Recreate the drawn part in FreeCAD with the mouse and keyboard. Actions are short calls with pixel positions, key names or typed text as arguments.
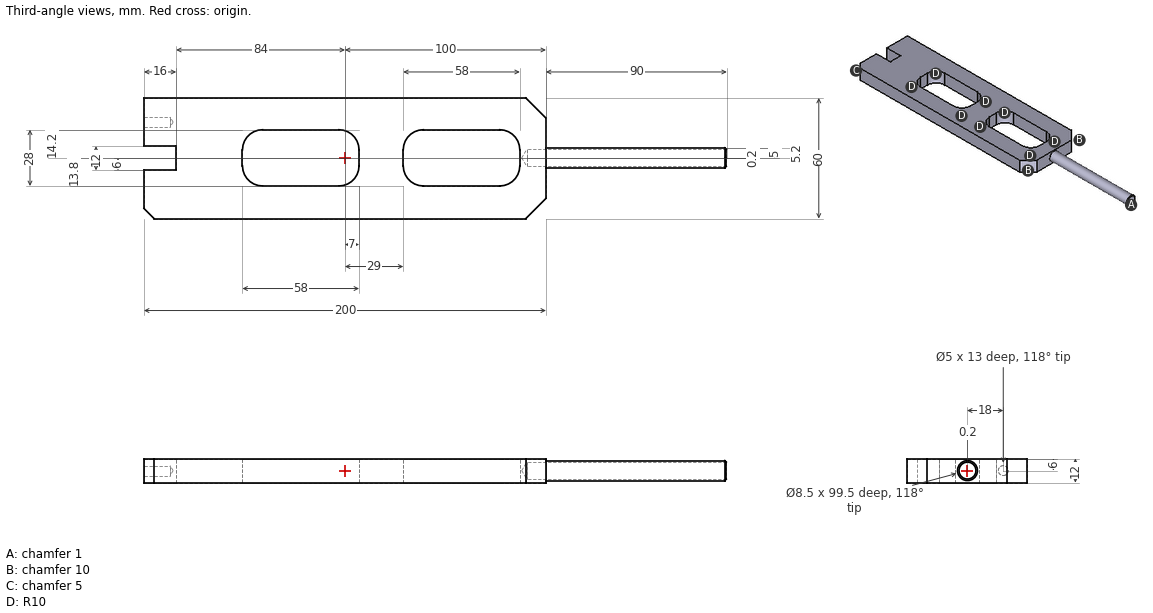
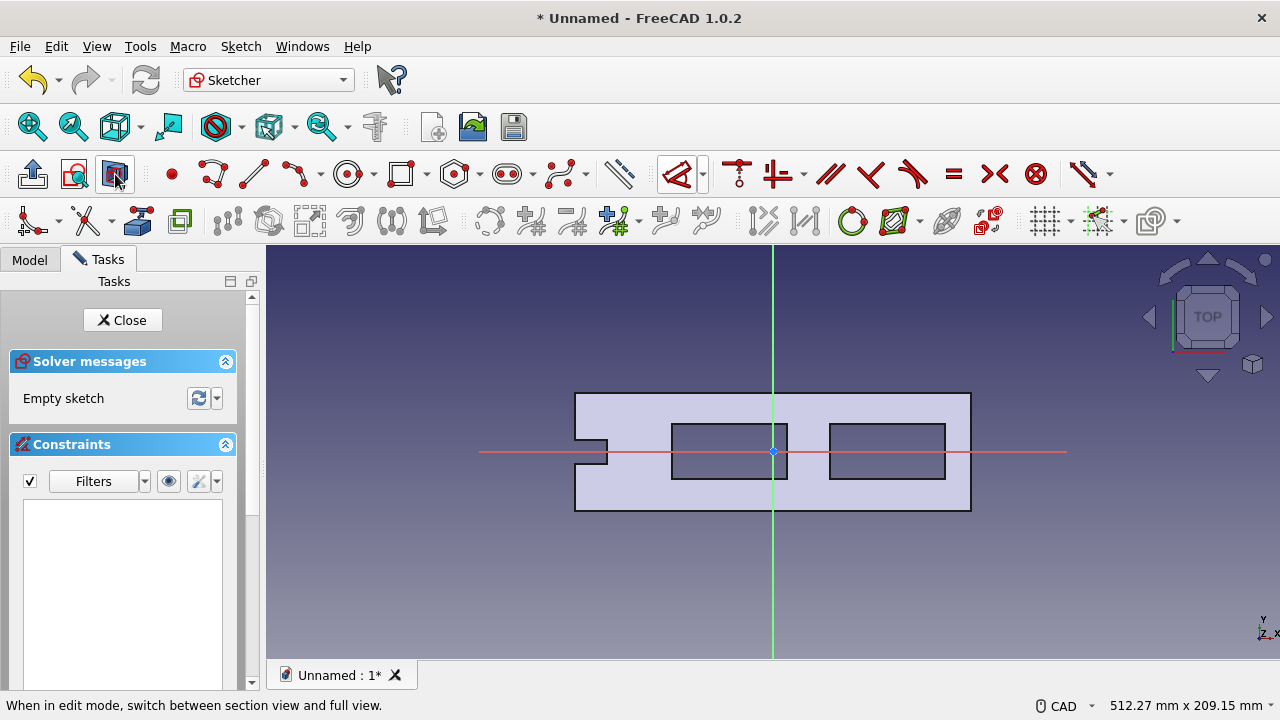
scroll(294, 475, down, 1)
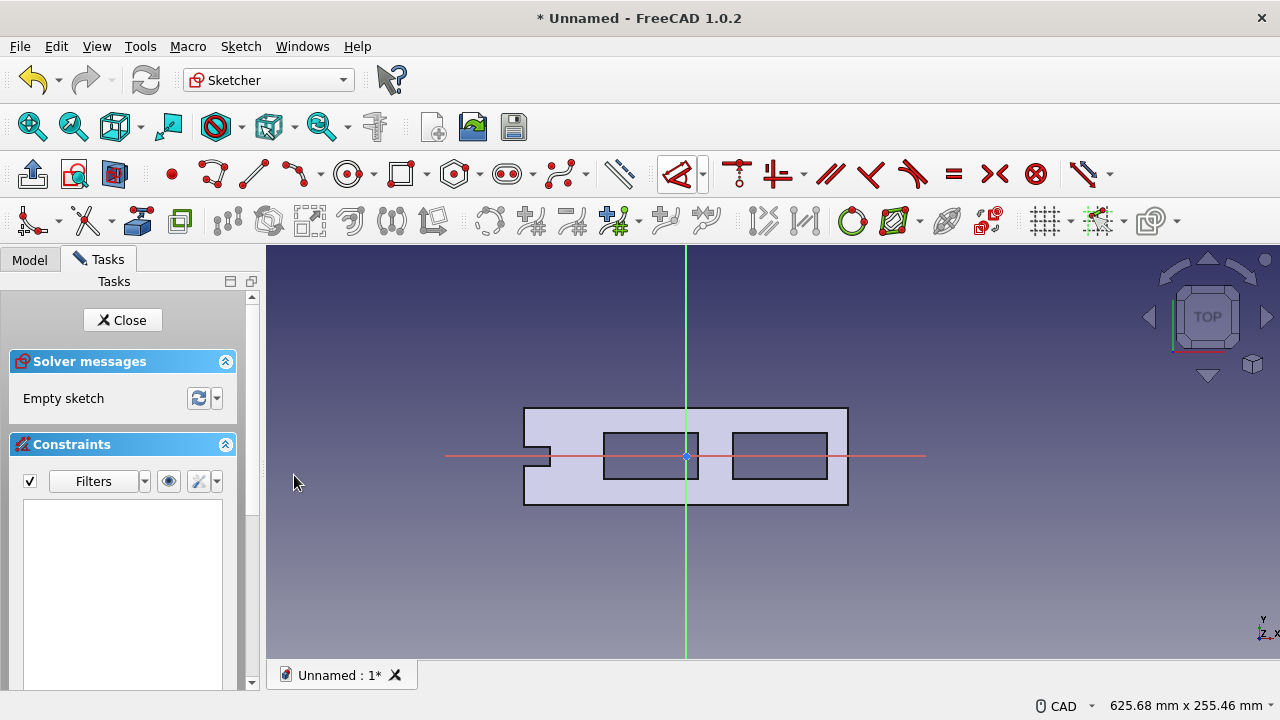
scroll(1005, 452, up, 3)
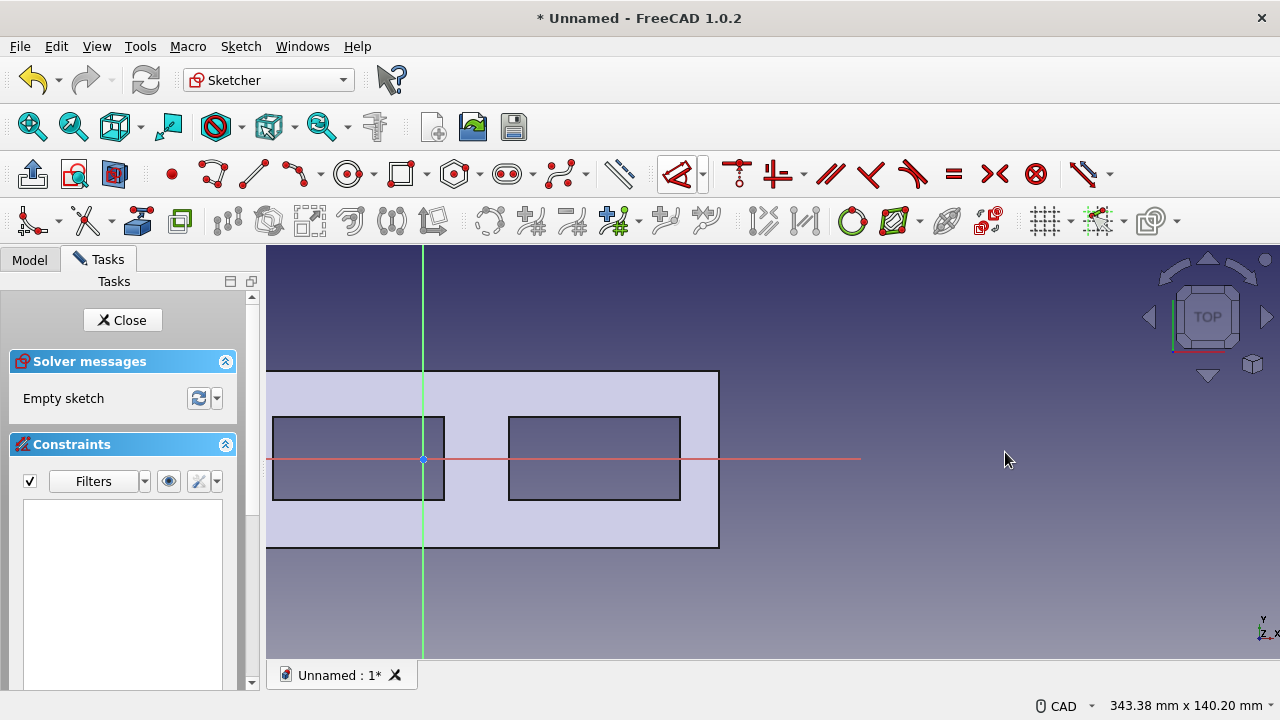
key(g)
key(r)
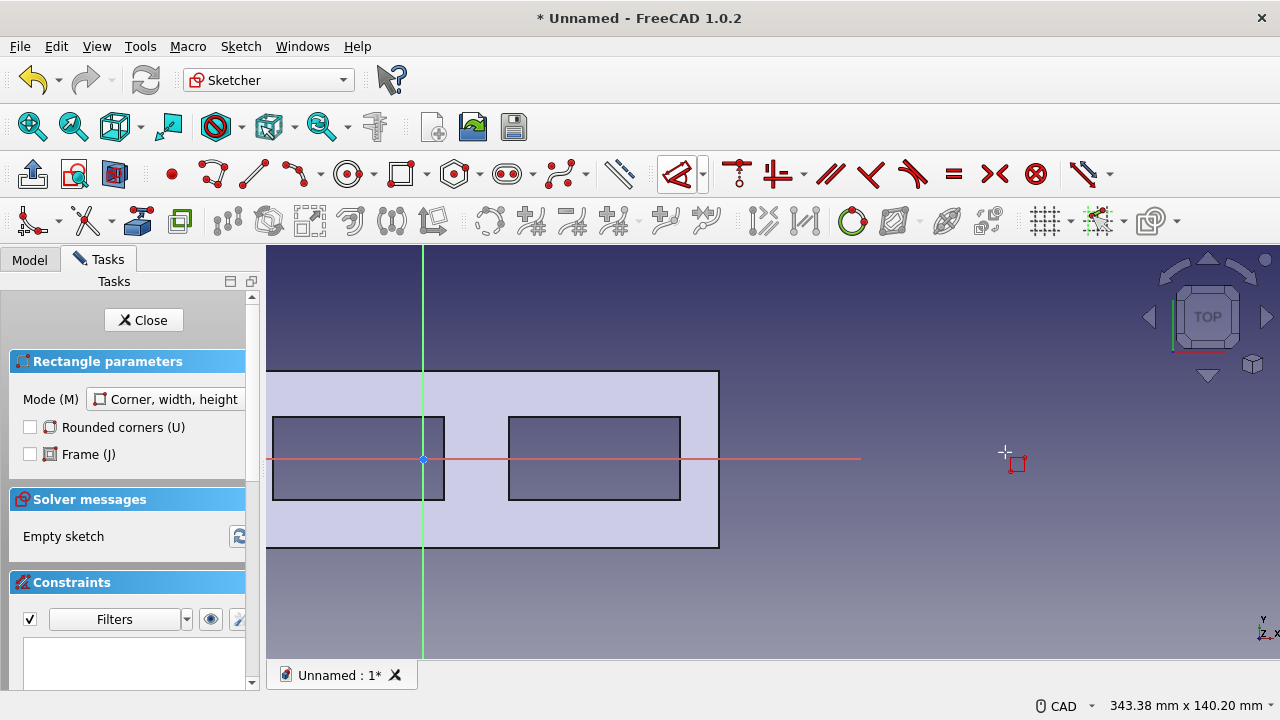
click(719, 444)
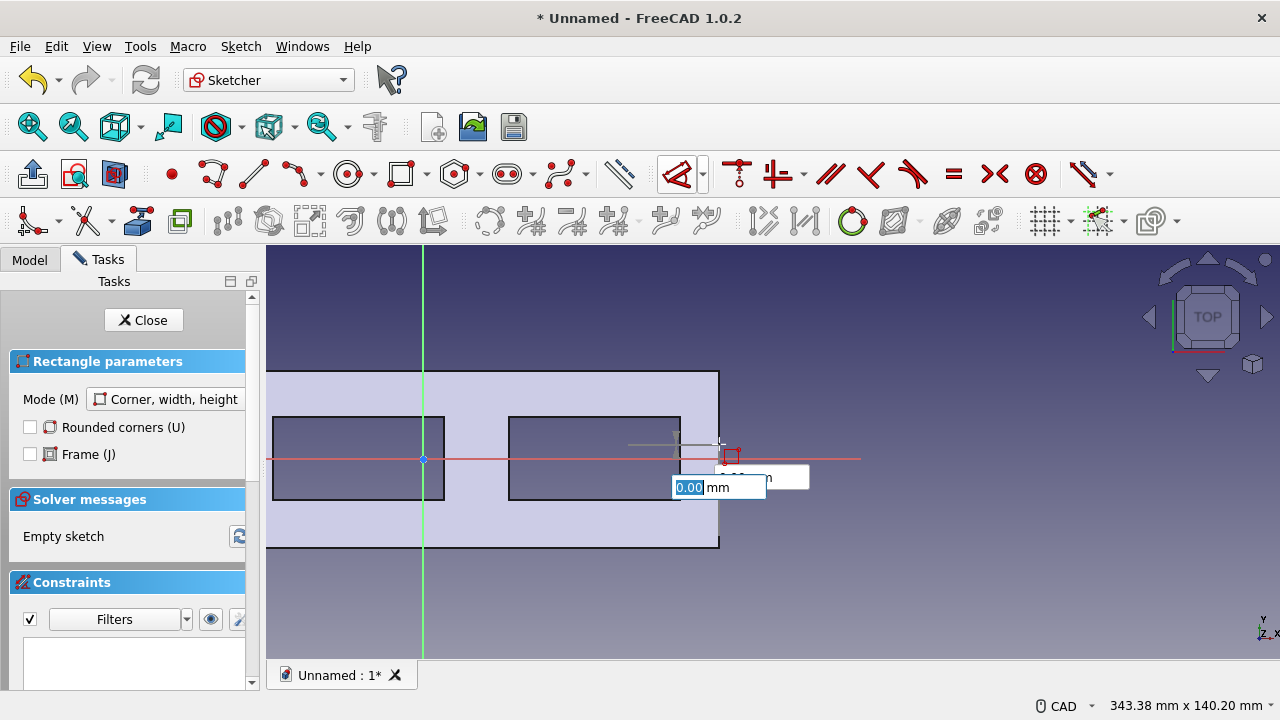
scroll(985, 459, up, 17)
move(950, 437)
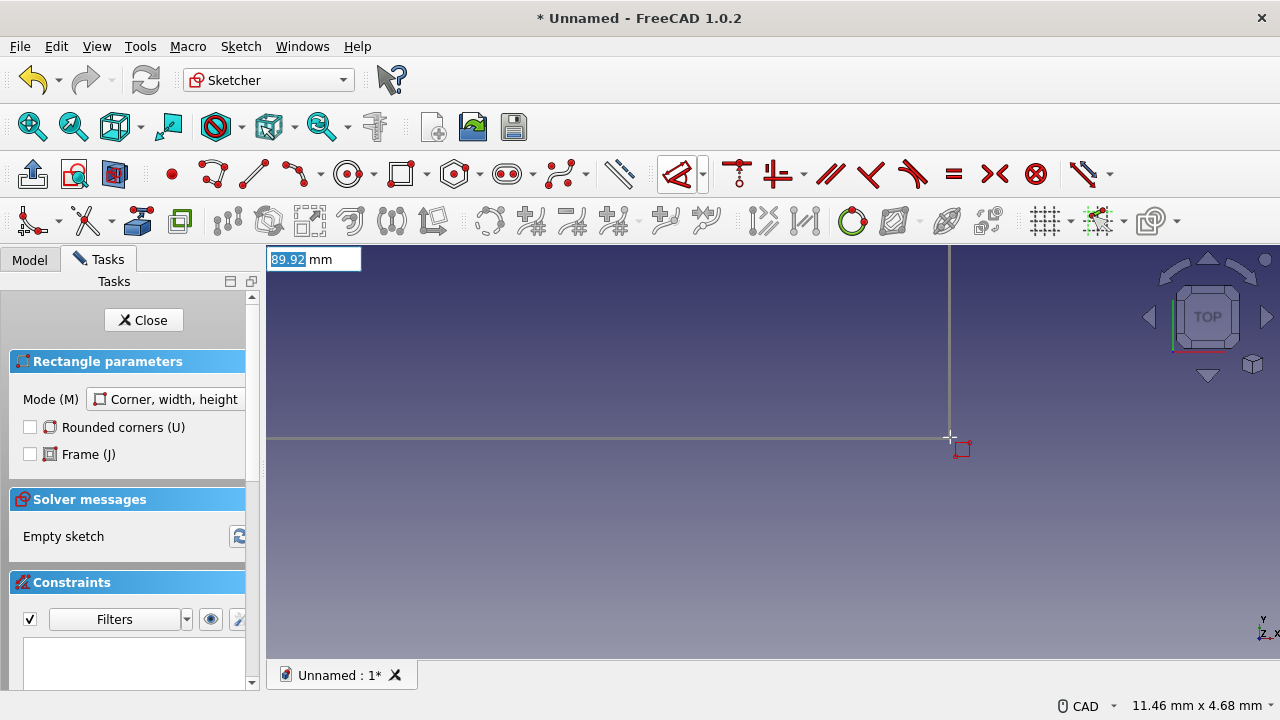
text(90)
key(Tab)
text(5)
key(Return)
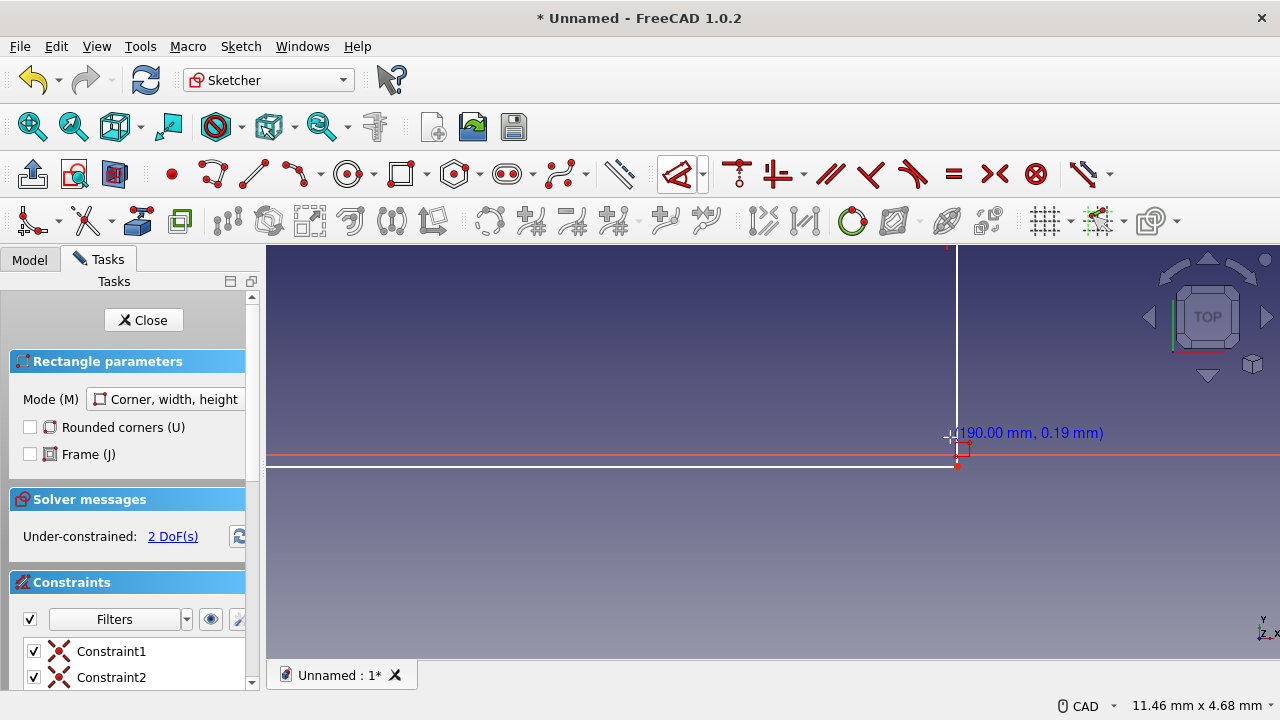
click(254, 174)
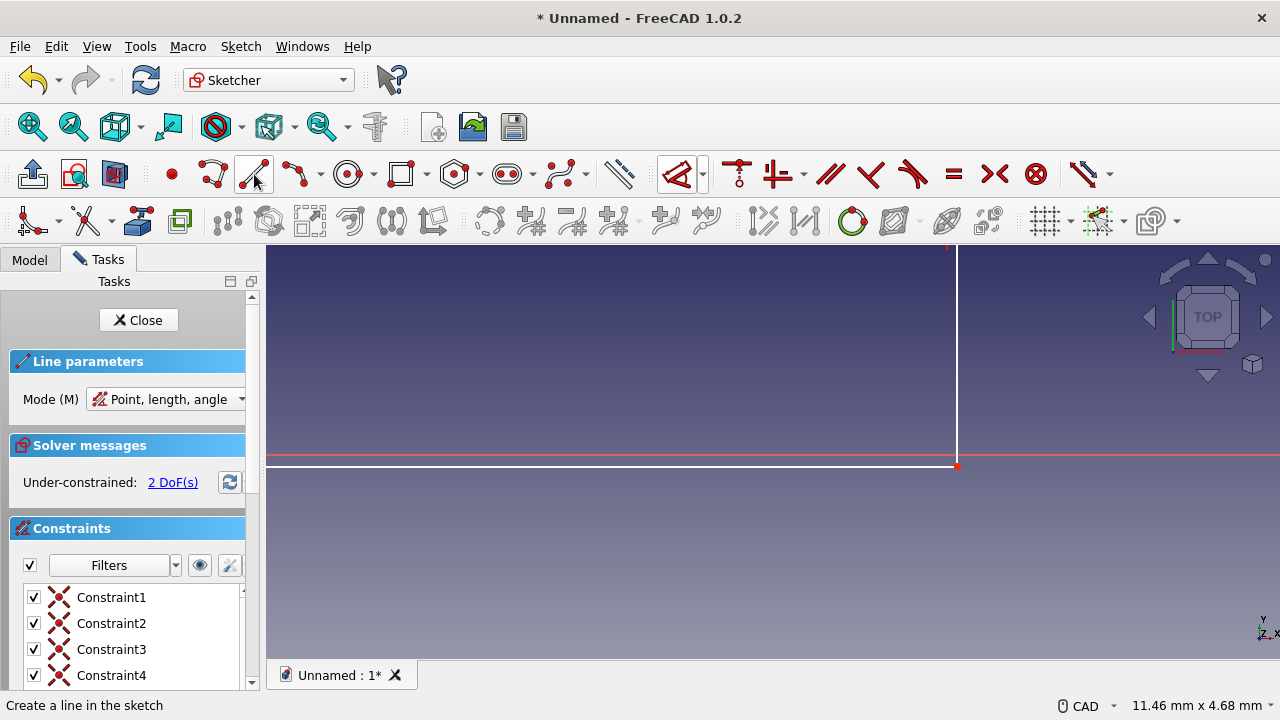
scroll(1051, 462, down, 16)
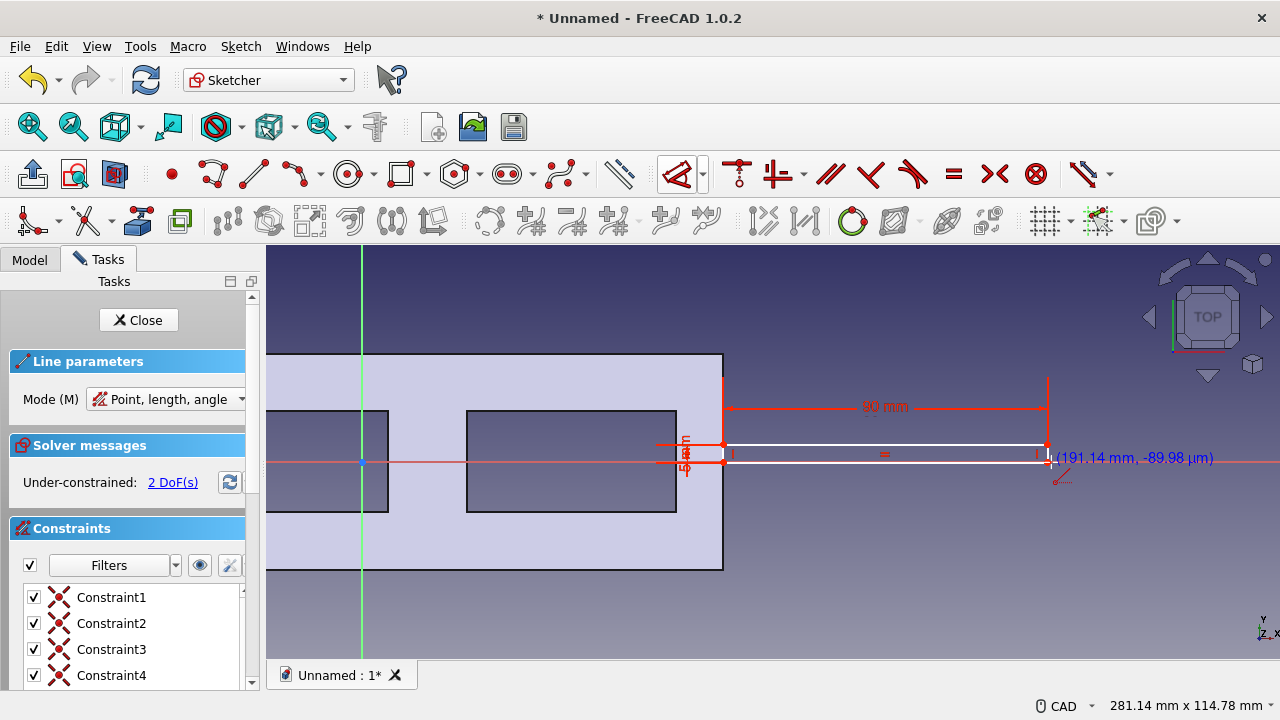
scroll(691, 461, up, 16)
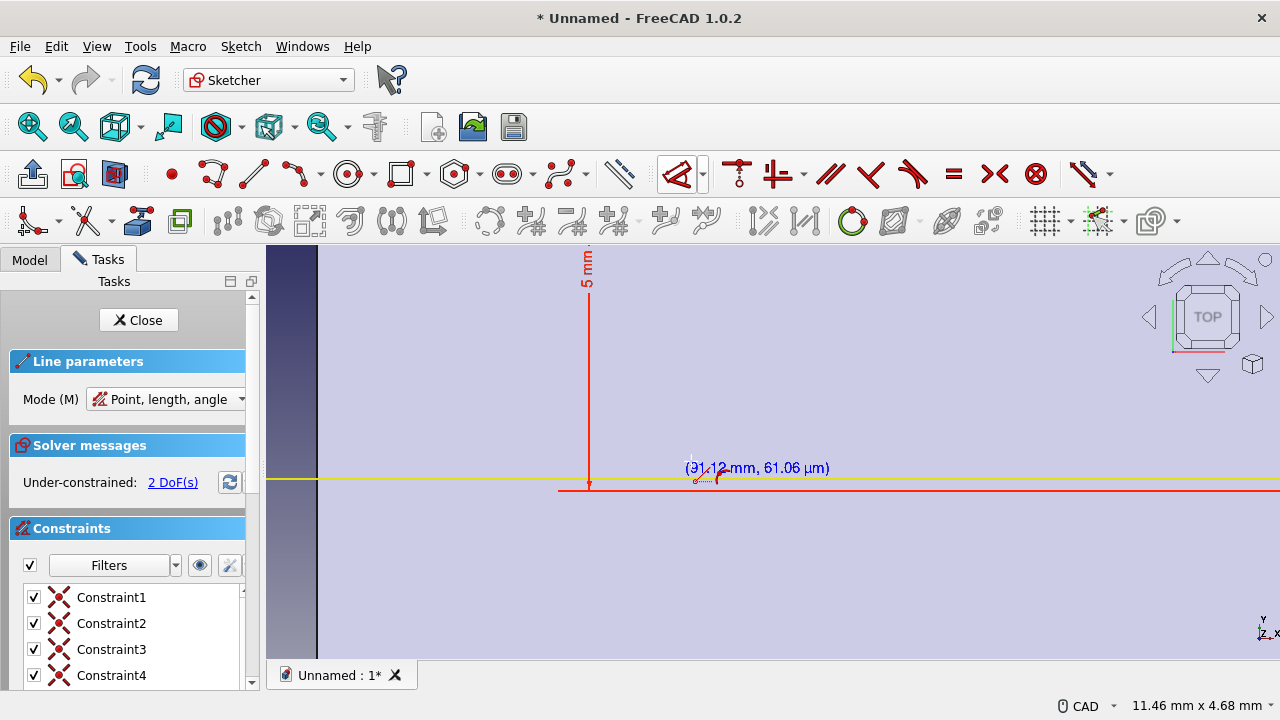
click(671, 461)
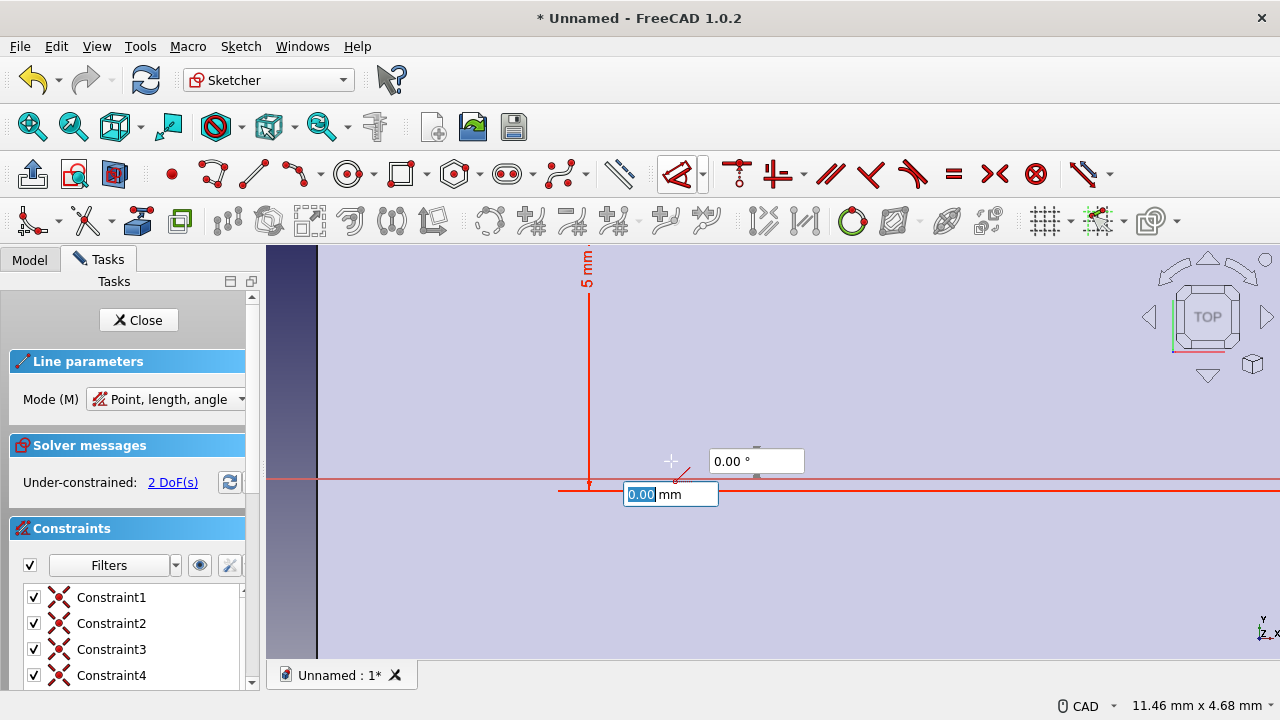
scroll(691, 461, down, 16)